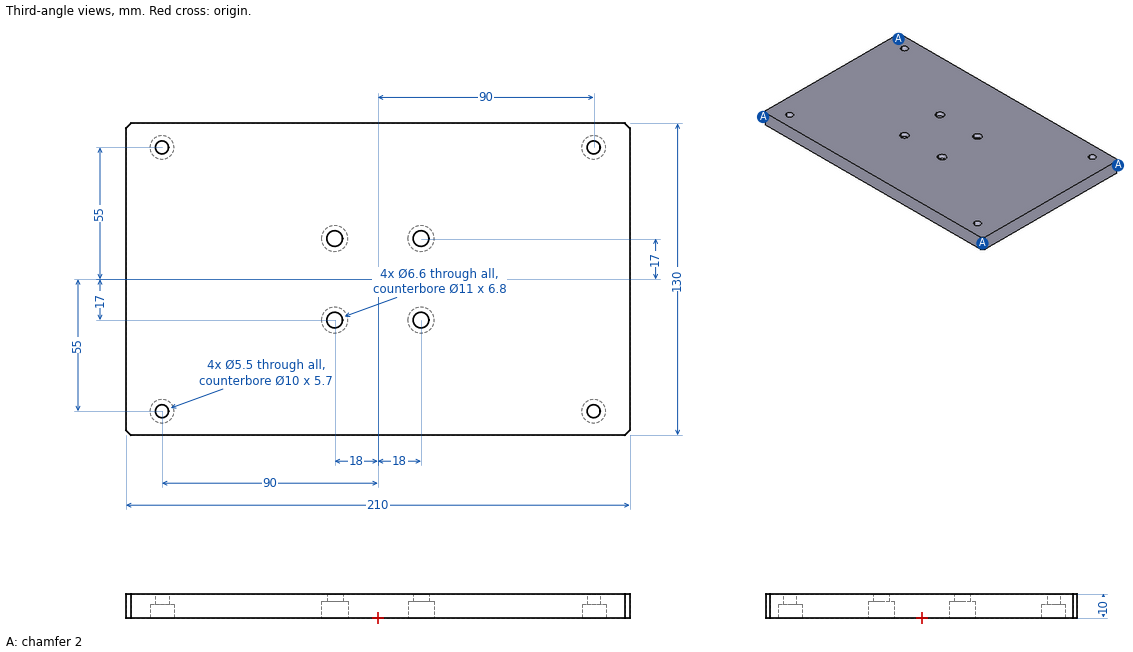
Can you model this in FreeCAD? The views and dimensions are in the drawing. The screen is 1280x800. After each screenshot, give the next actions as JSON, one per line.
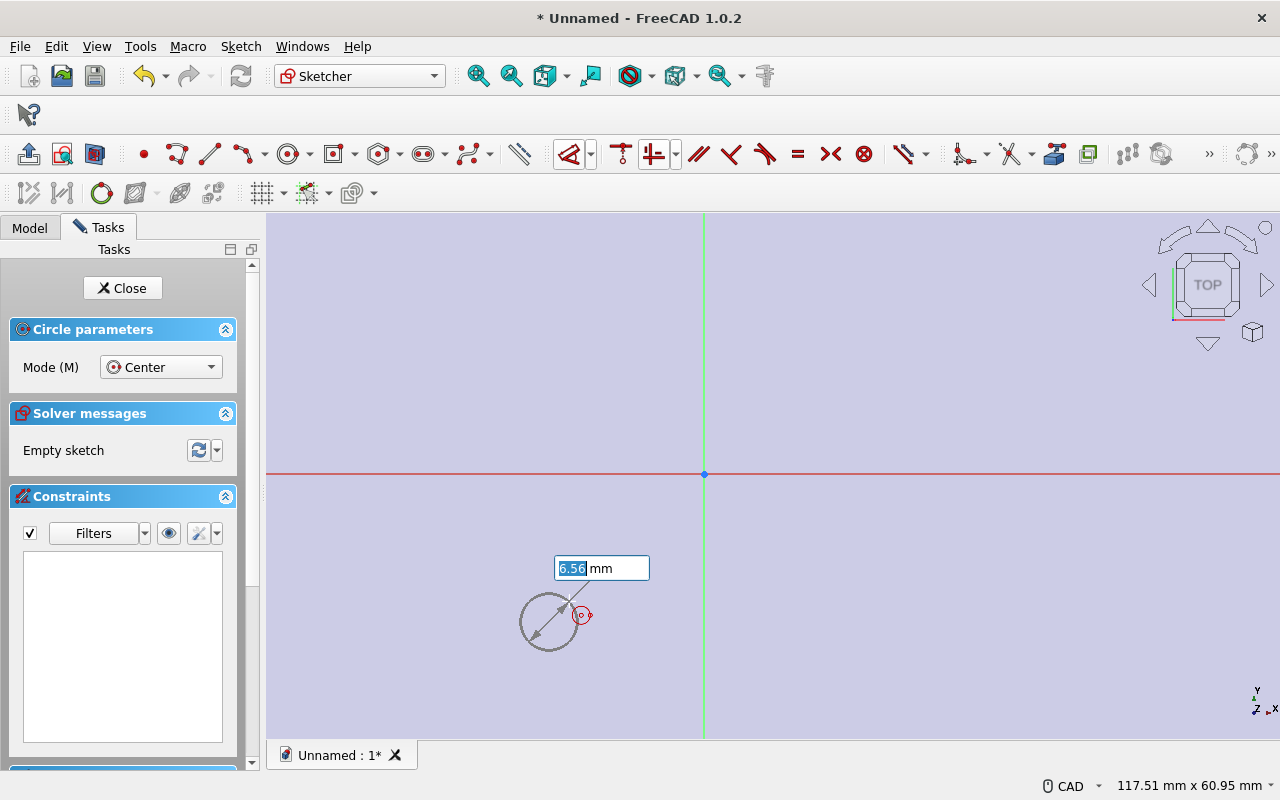
{"action": "type", "text": "6.6"}
{"action": "key", "text": "Return"}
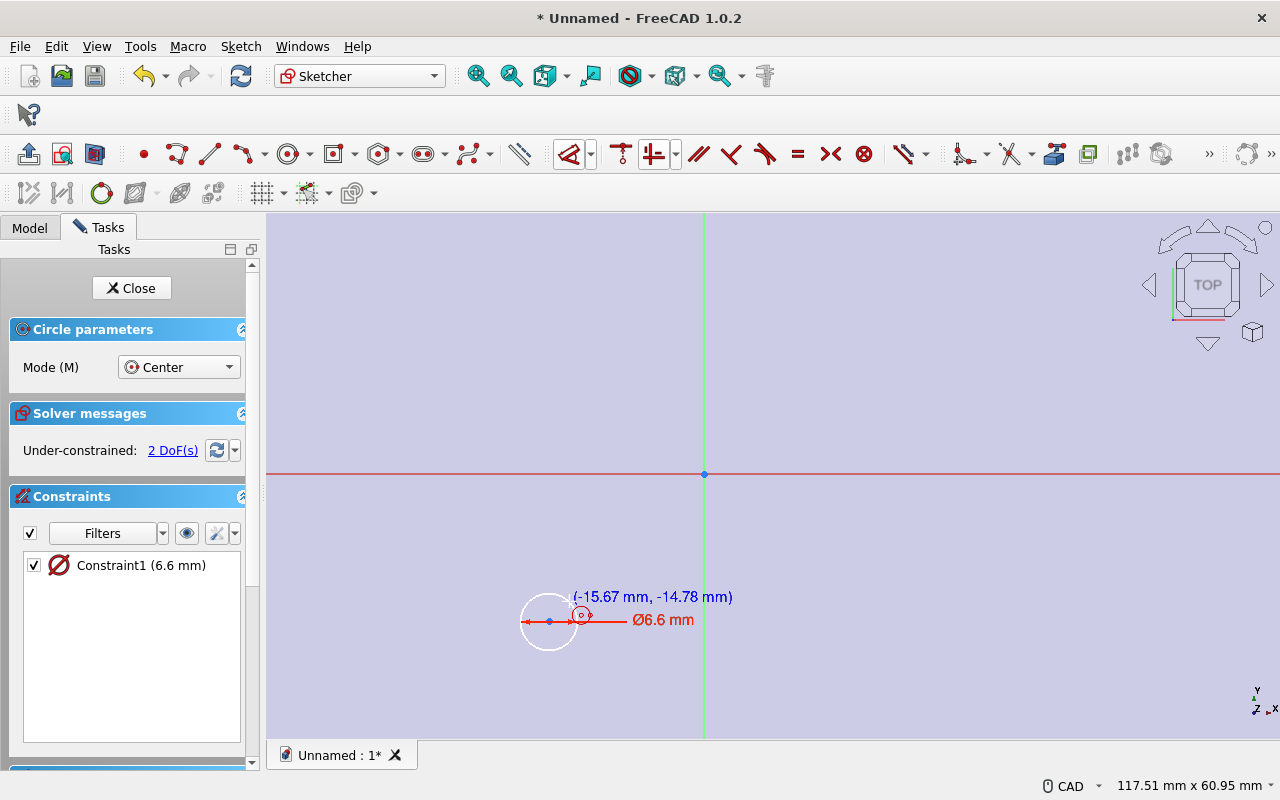
{"action": "left_click", "coordinate": [860, 621]}
{"action": "mouse_move", "coordinate": [880, 601]}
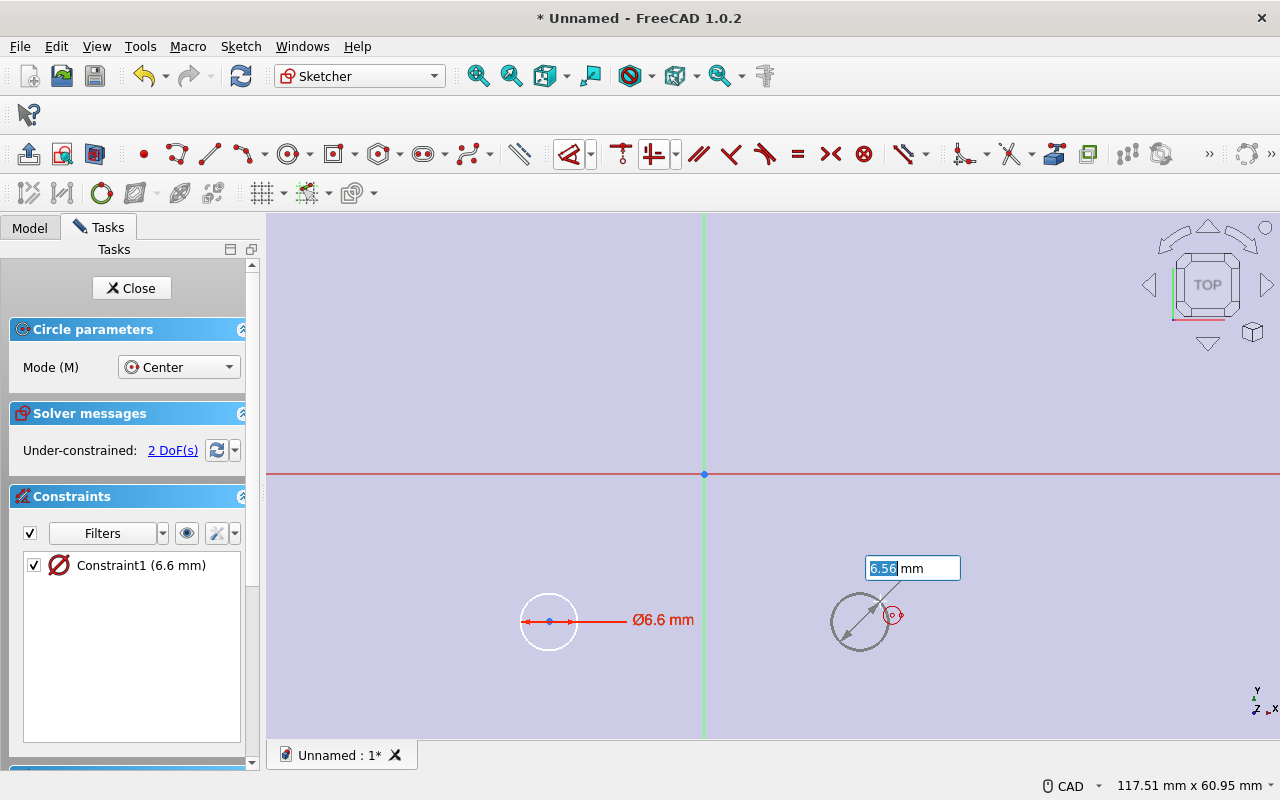
{"action": "type", "text": "6.6"}
{"action": "key", "text": "Return"}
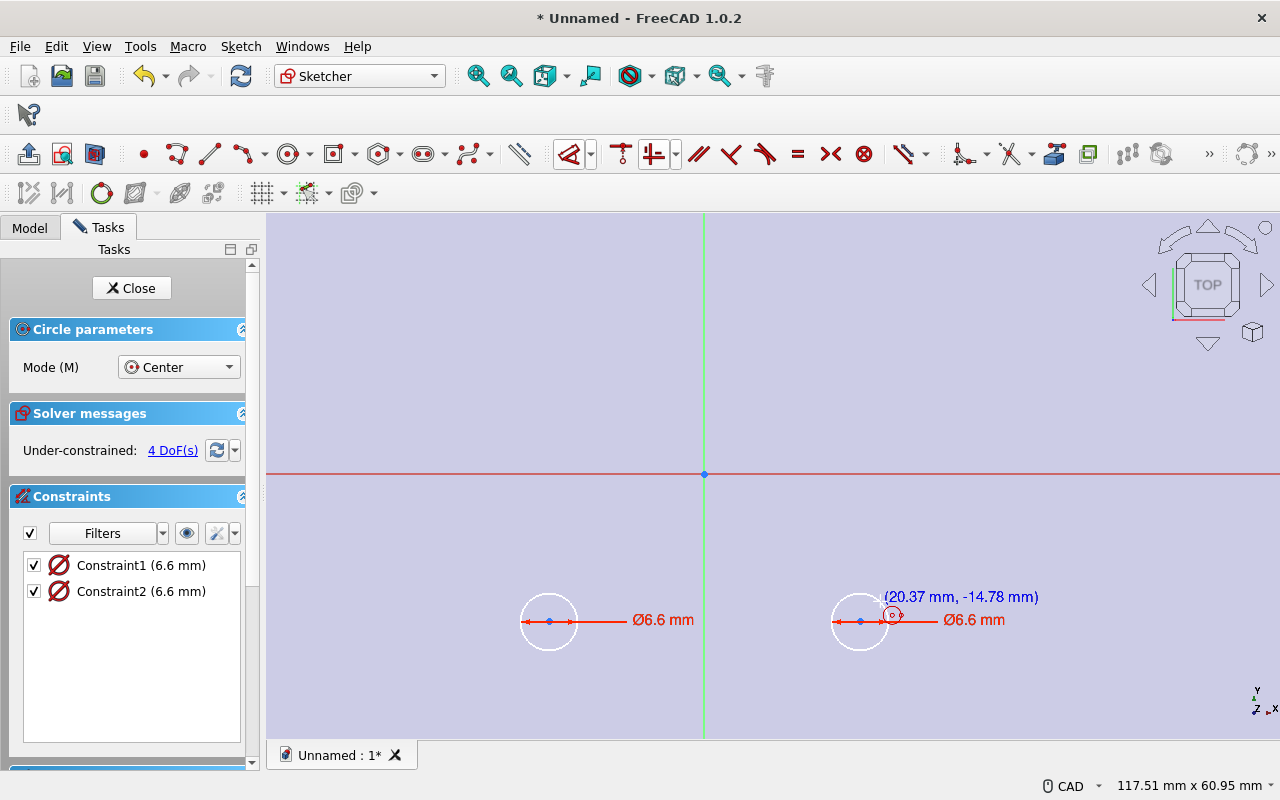
{"action": "left_click", "coordinate": [860, 328]}
{"action": "mouse_move", "coordinate": [880, 308]}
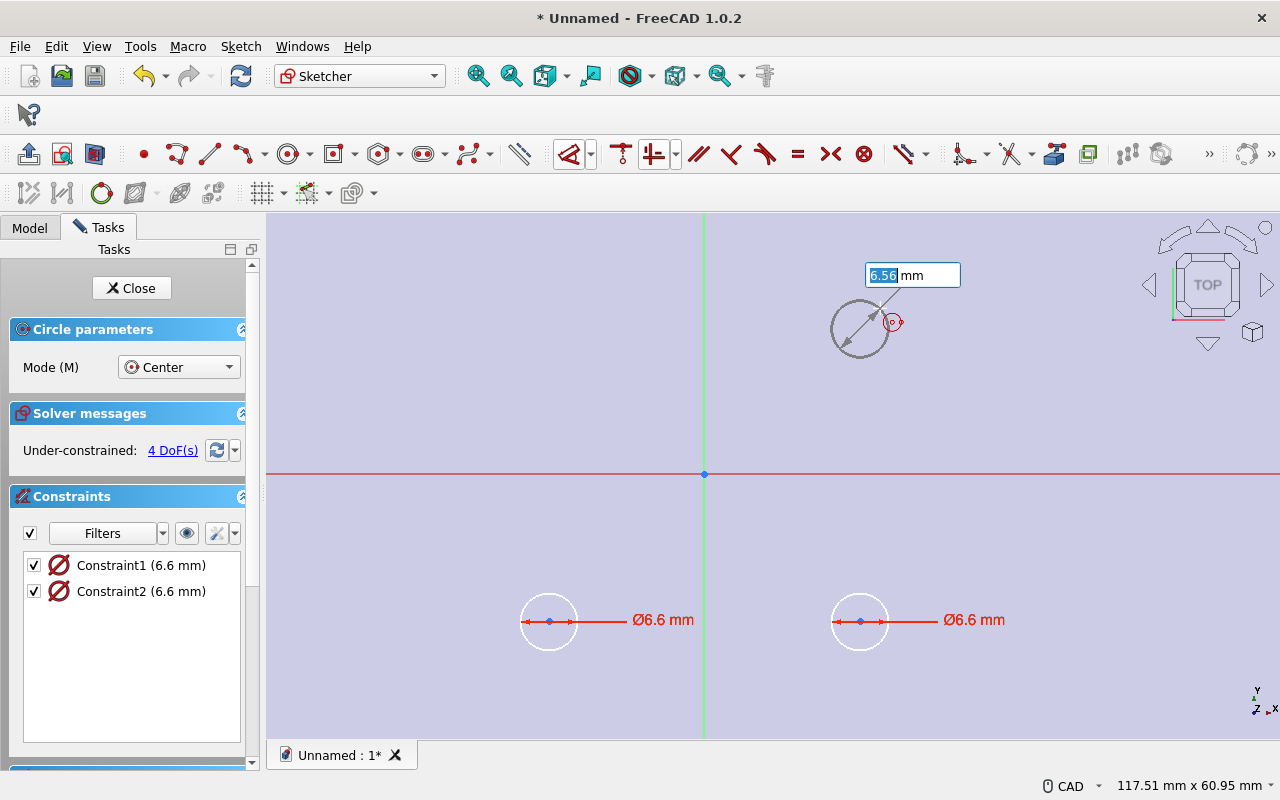
{"action": "type", "text": "6.6"}
{"action": "key", "text": "Return"}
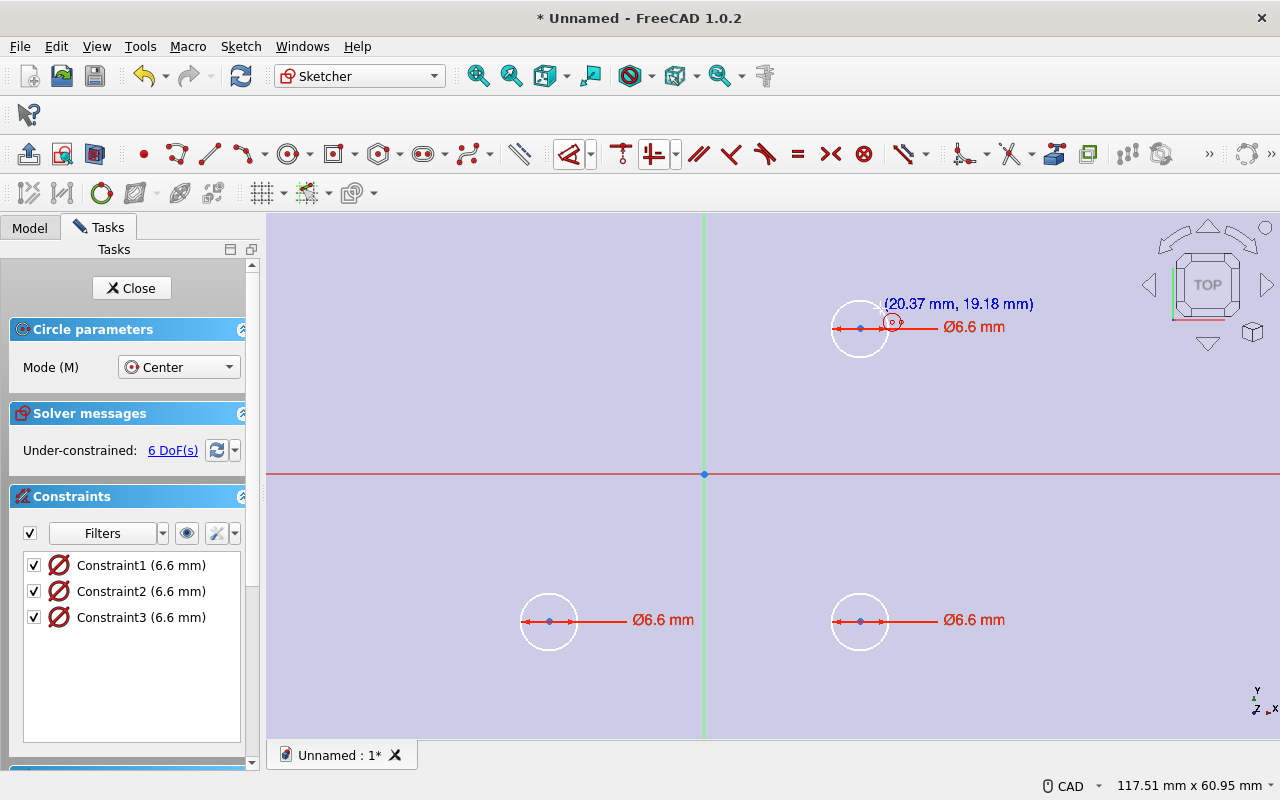
{"action": "left_click", "coordinate": [549, 328]}
{"action": "mouse_move", "coordinate": [569, 308]}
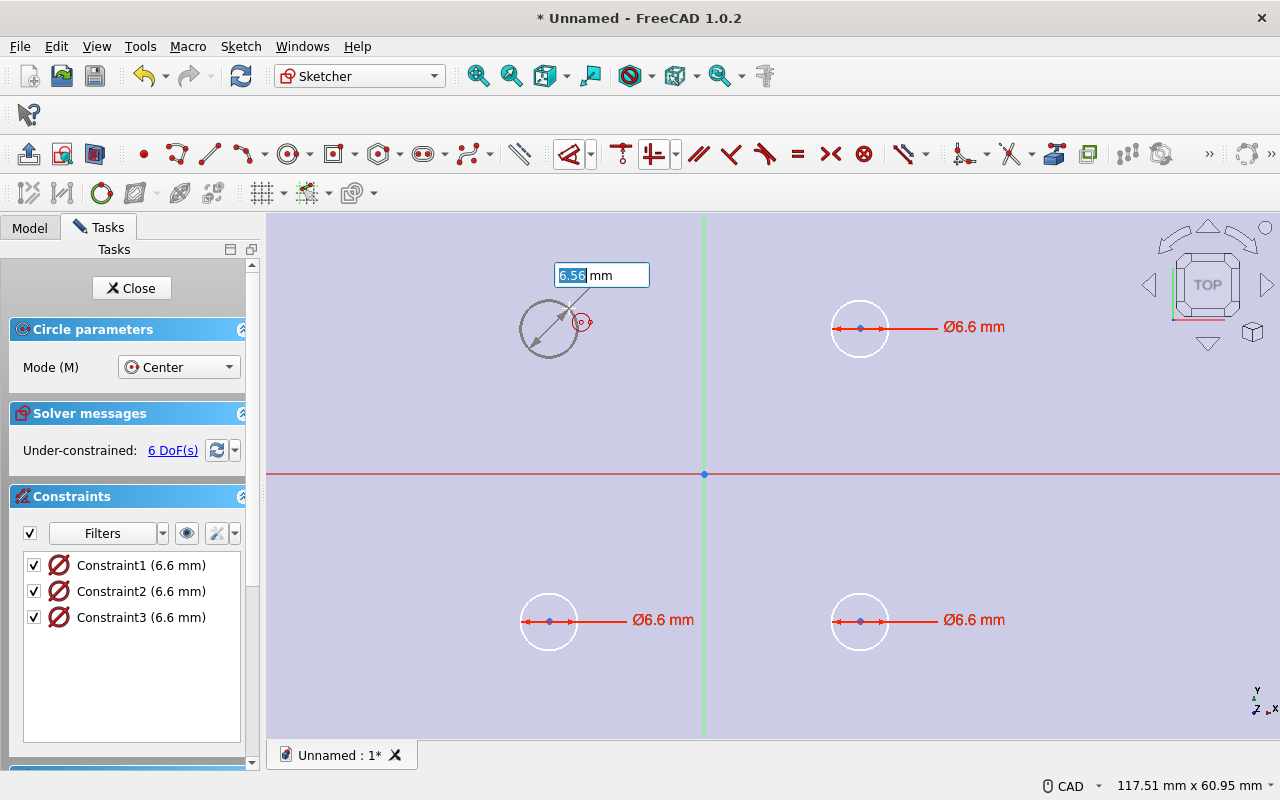
{"action": "type", "text": "6.6"}
{"action": "key", "text": "Return"}
{"action": "key", "text": "Escape"}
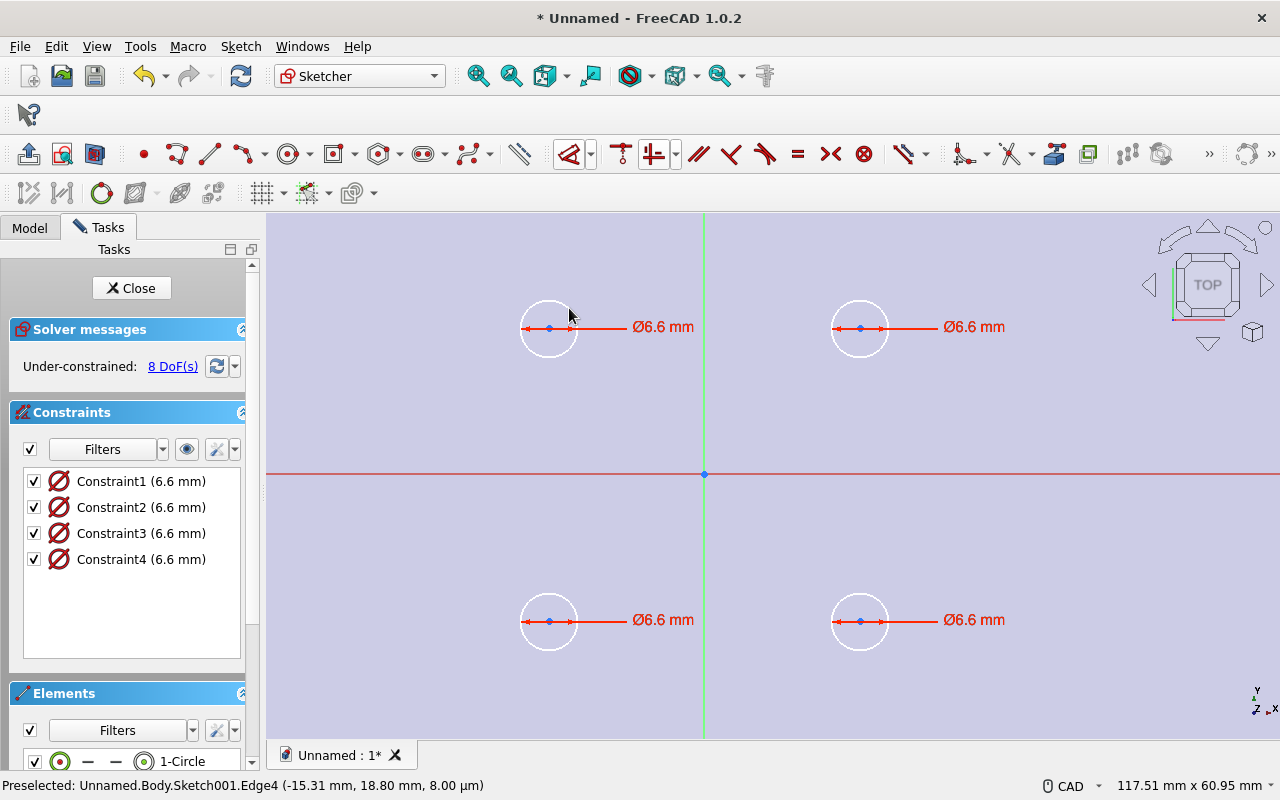
{"action": "left_click", "coordinate": [549, 622]}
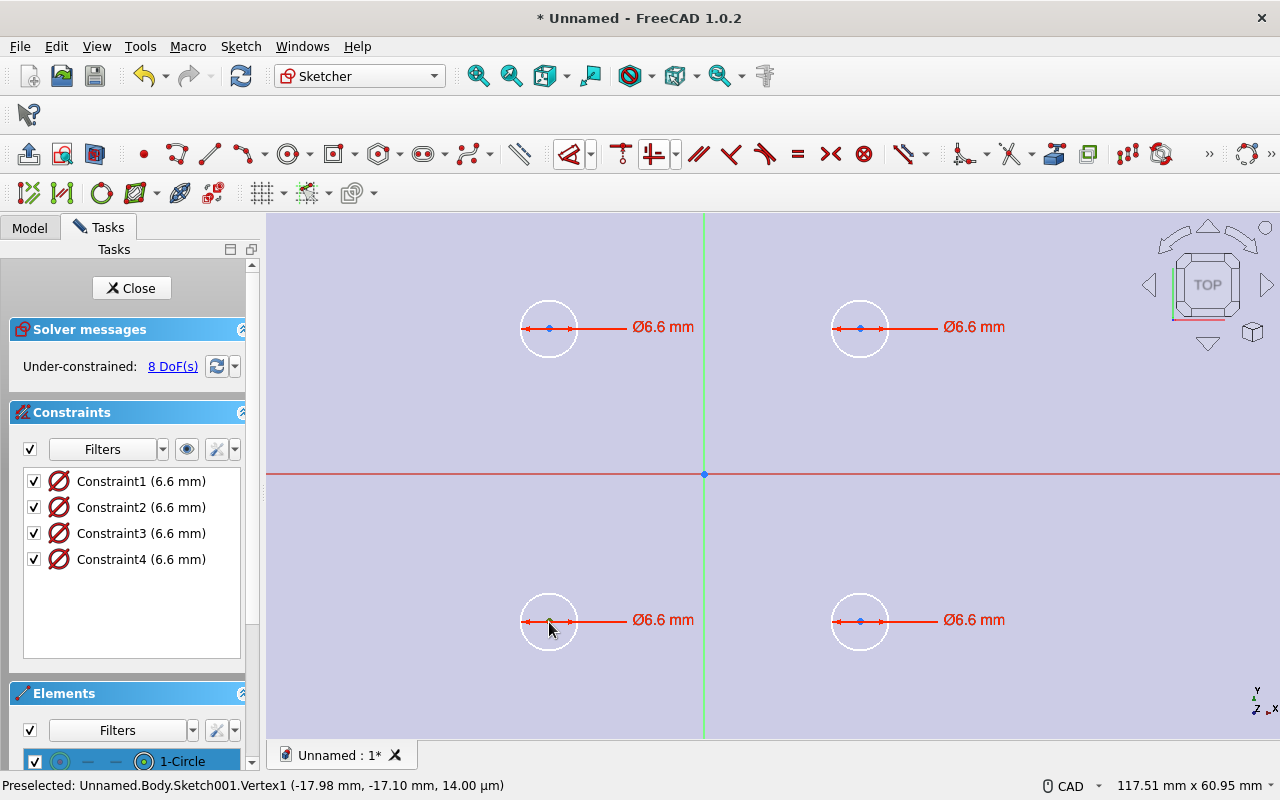
{"action": "left_click", "coordinate": [860, 622]}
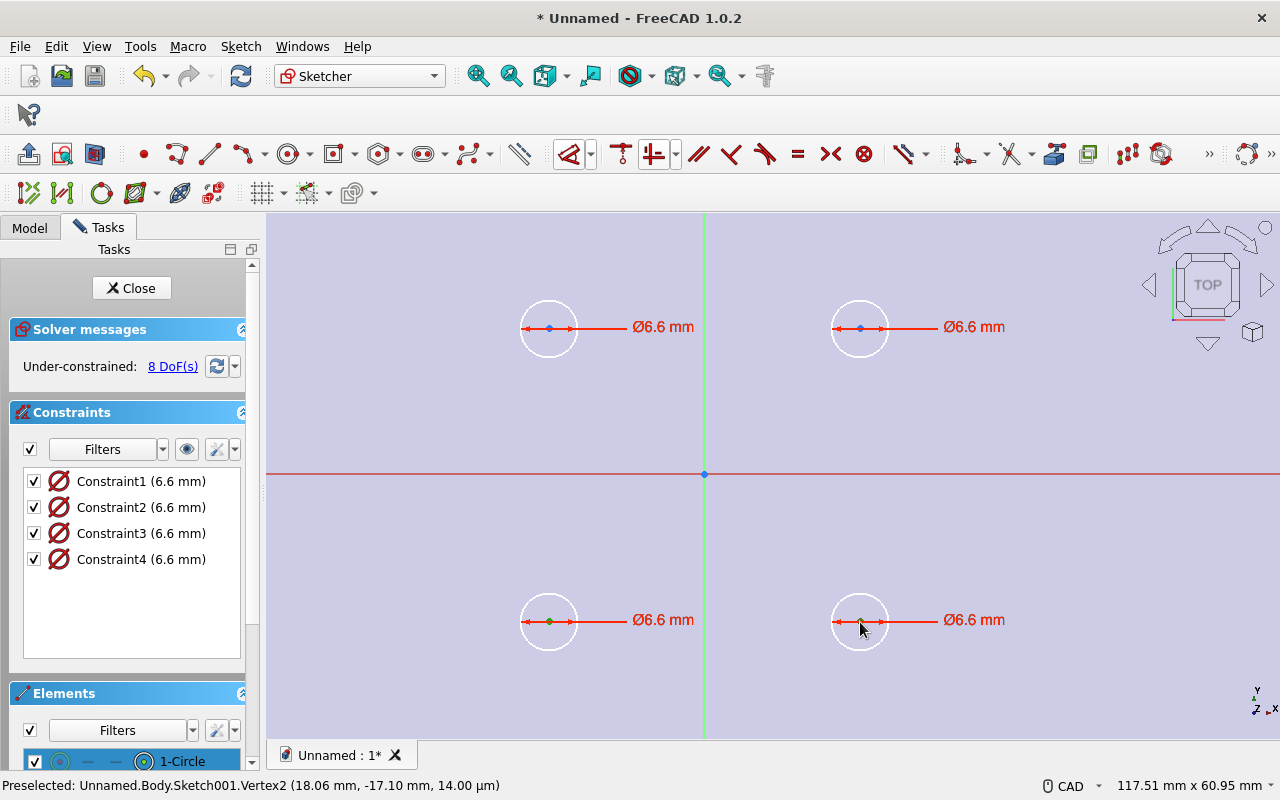
{"action": "key", "text": "h"}